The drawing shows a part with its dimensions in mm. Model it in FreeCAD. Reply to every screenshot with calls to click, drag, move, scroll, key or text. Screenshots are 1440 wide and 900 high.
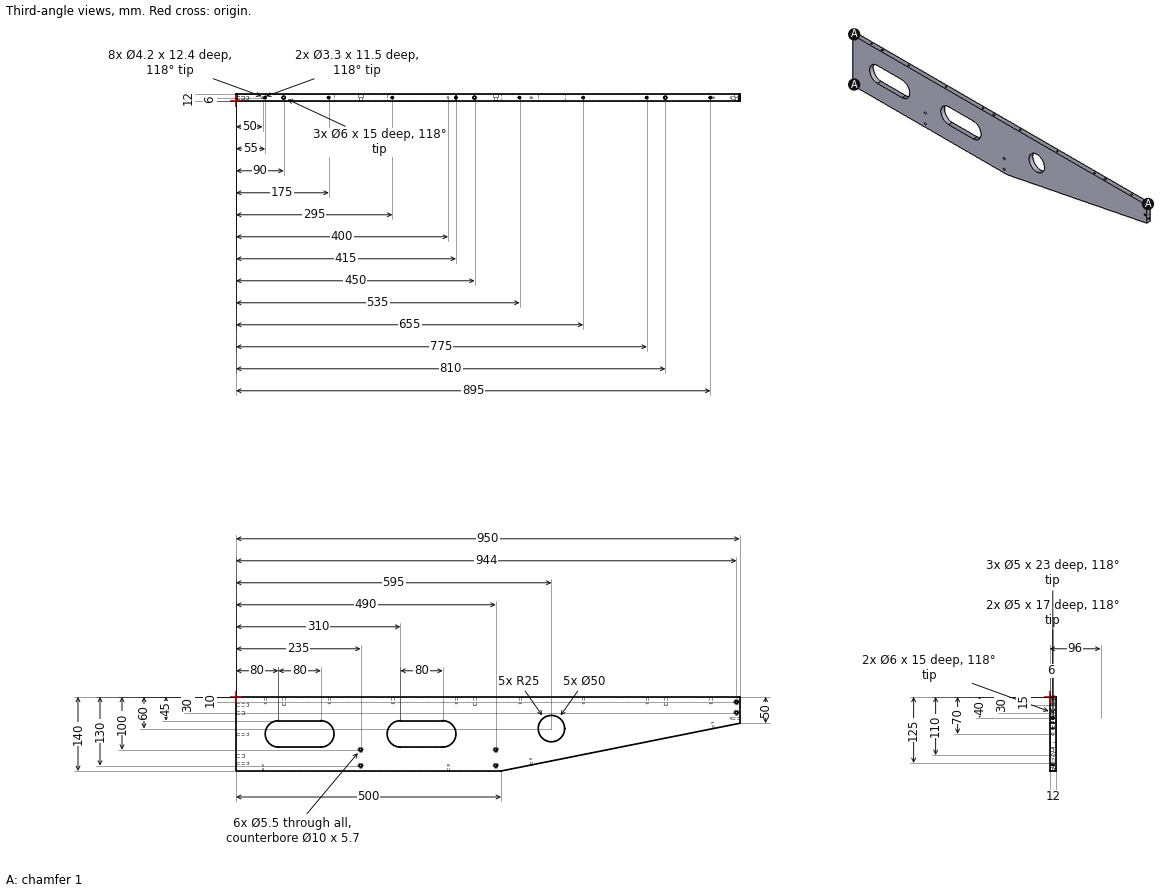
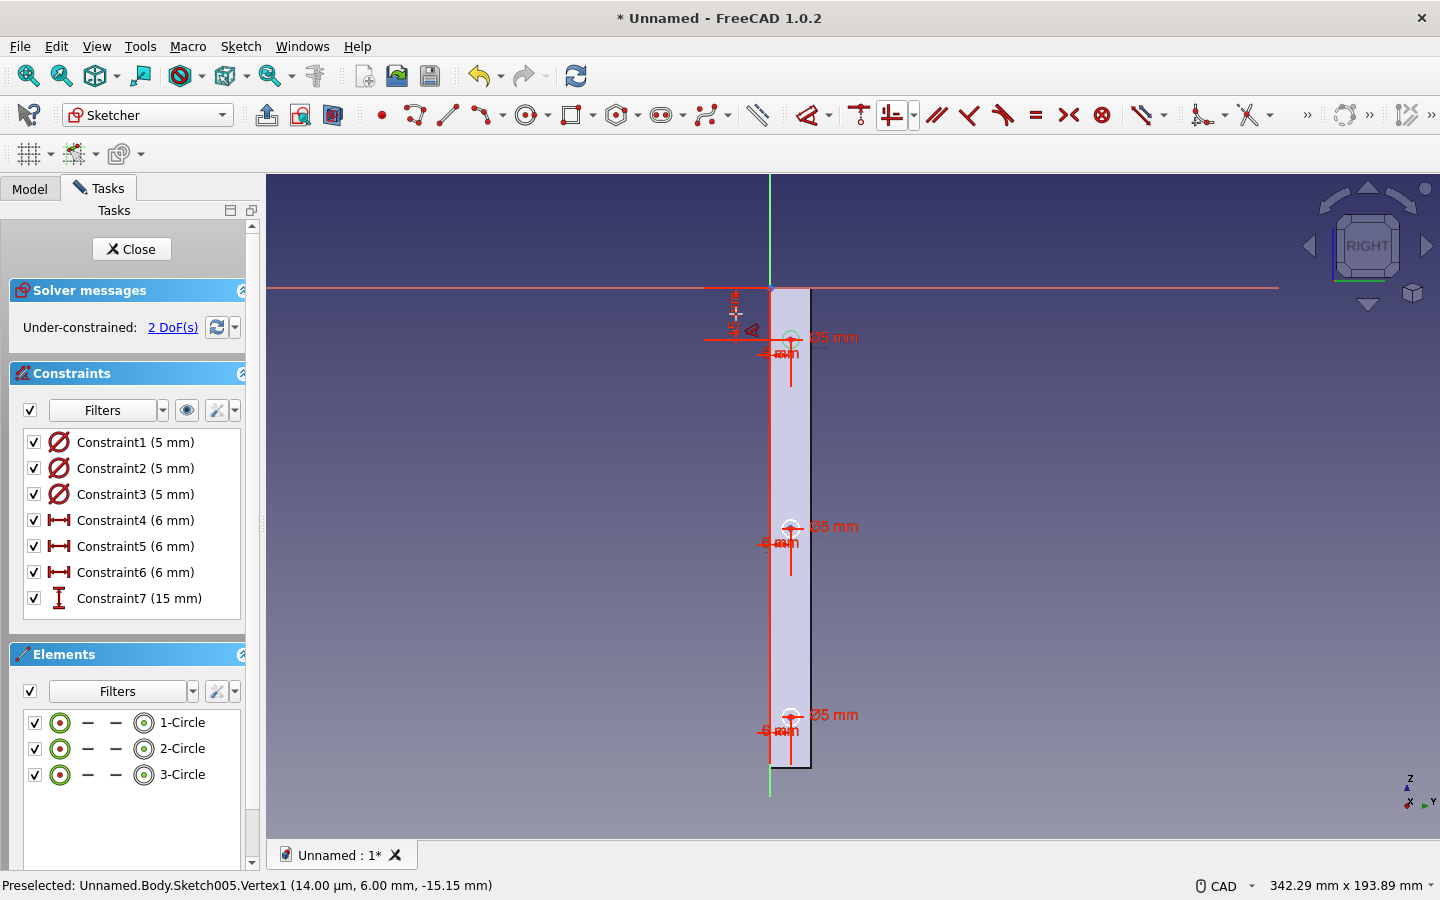
click(791, 529)
click(736, 408)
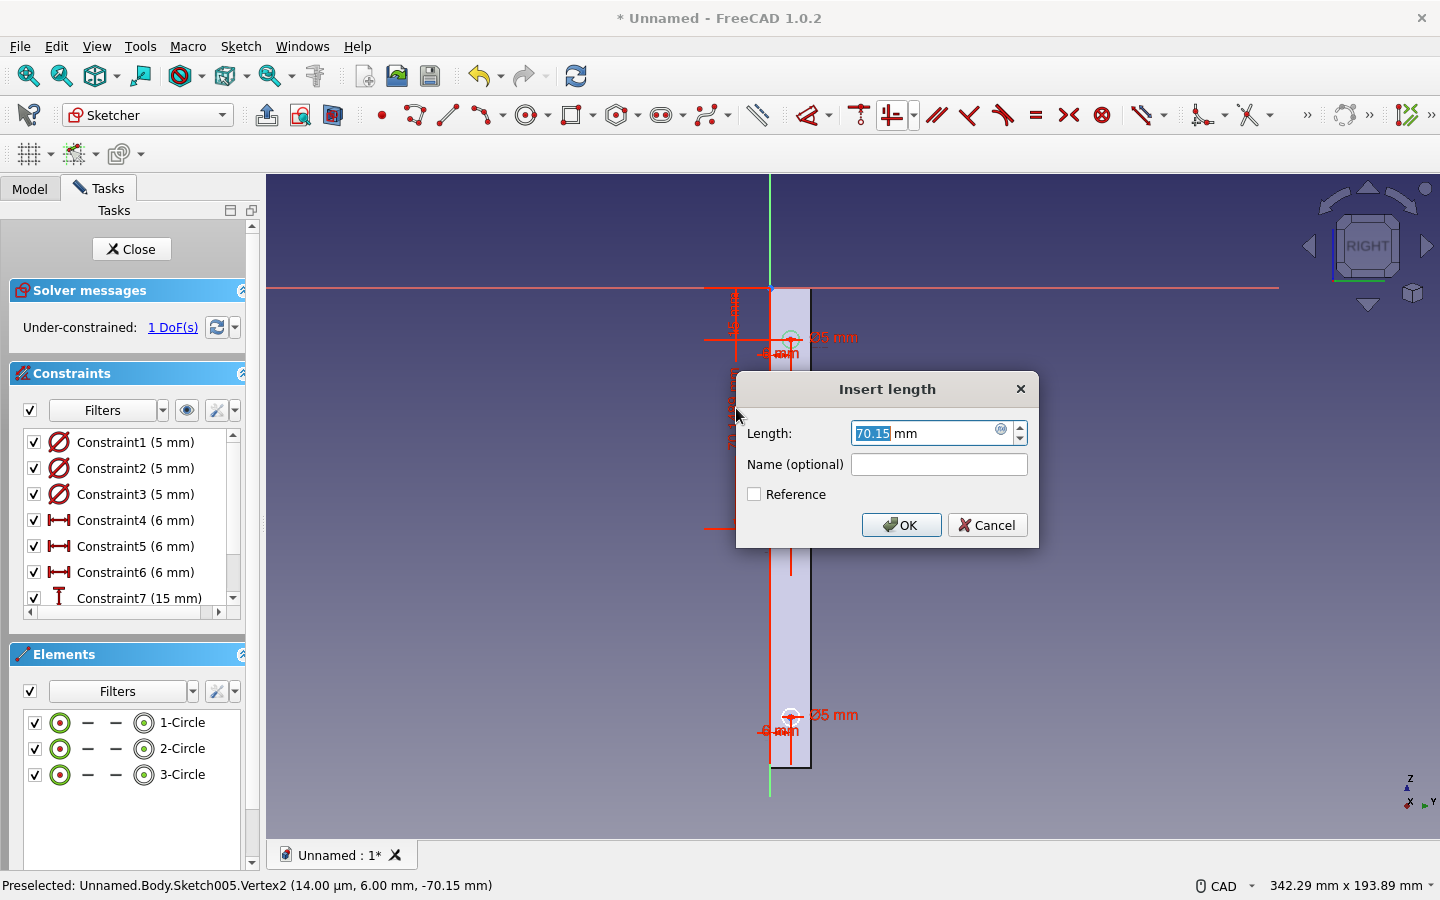
text(70)
key(Return)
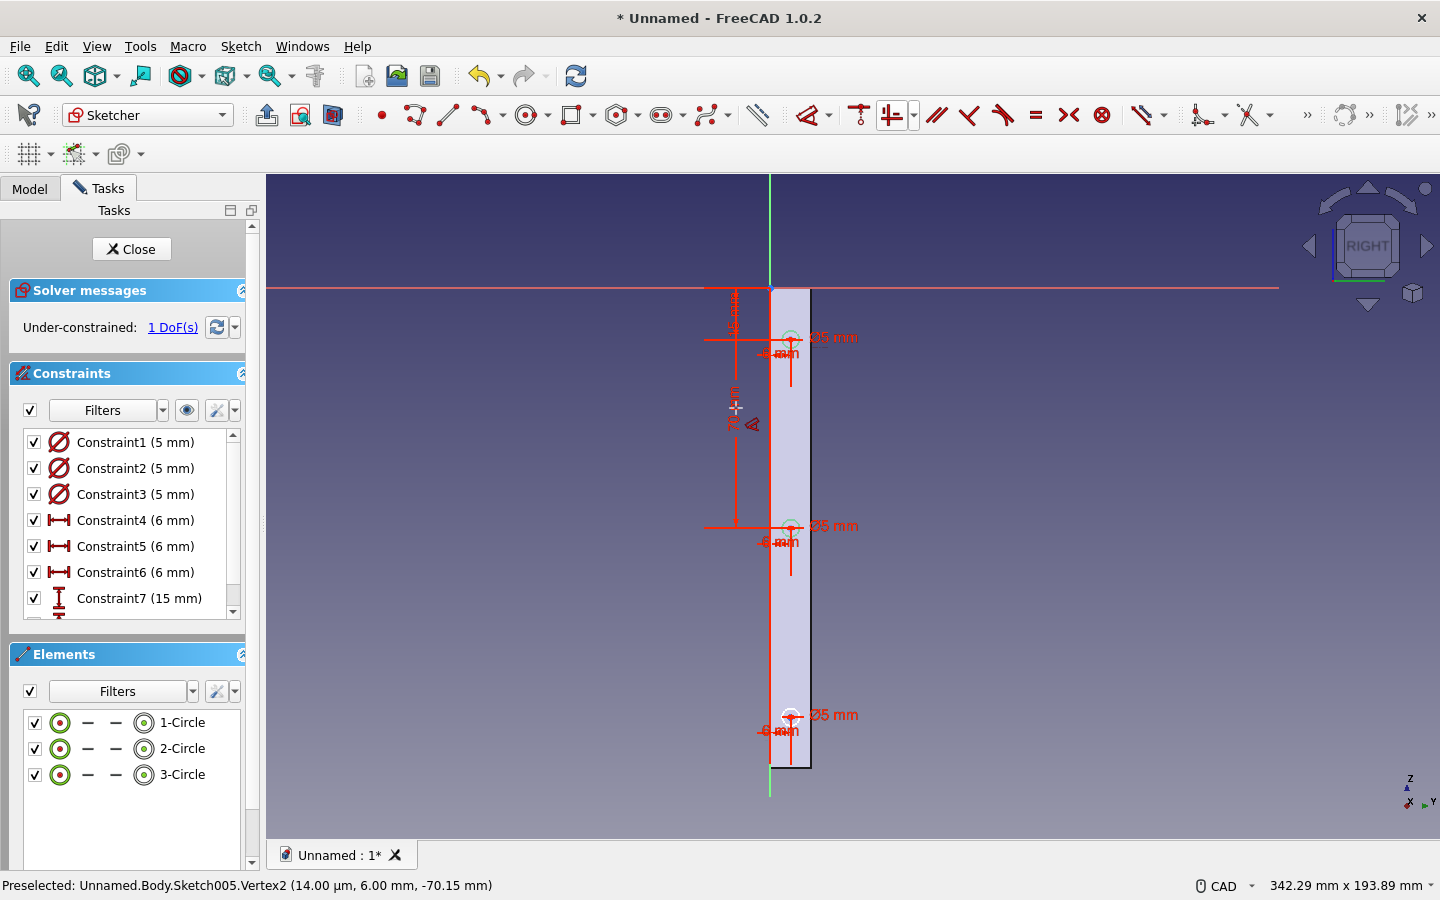
click(791, 717)
click(736, 503)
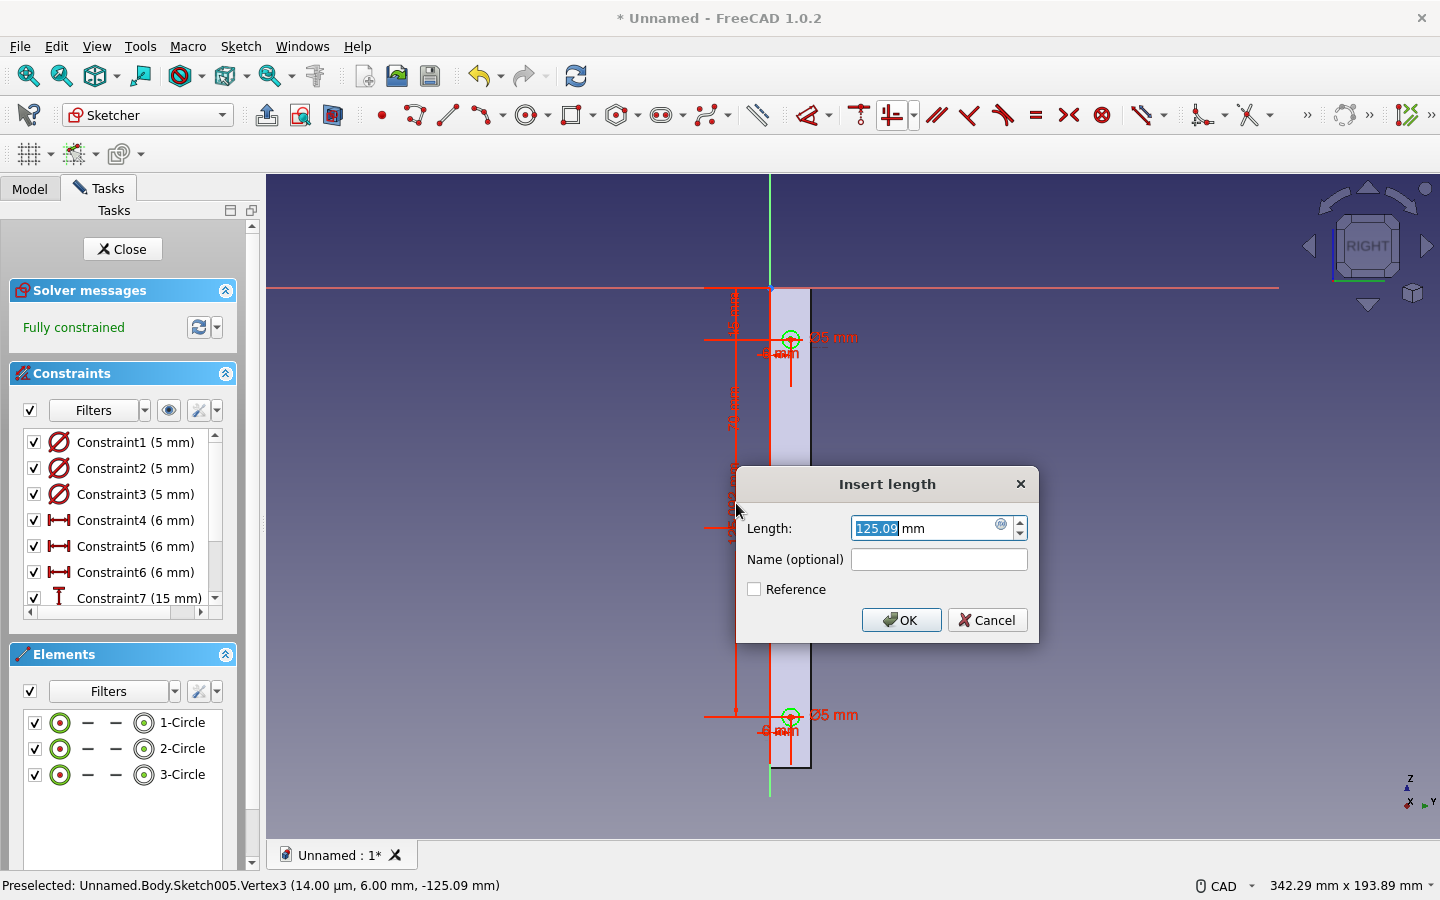
text(125)
key(Return)
key(Escape)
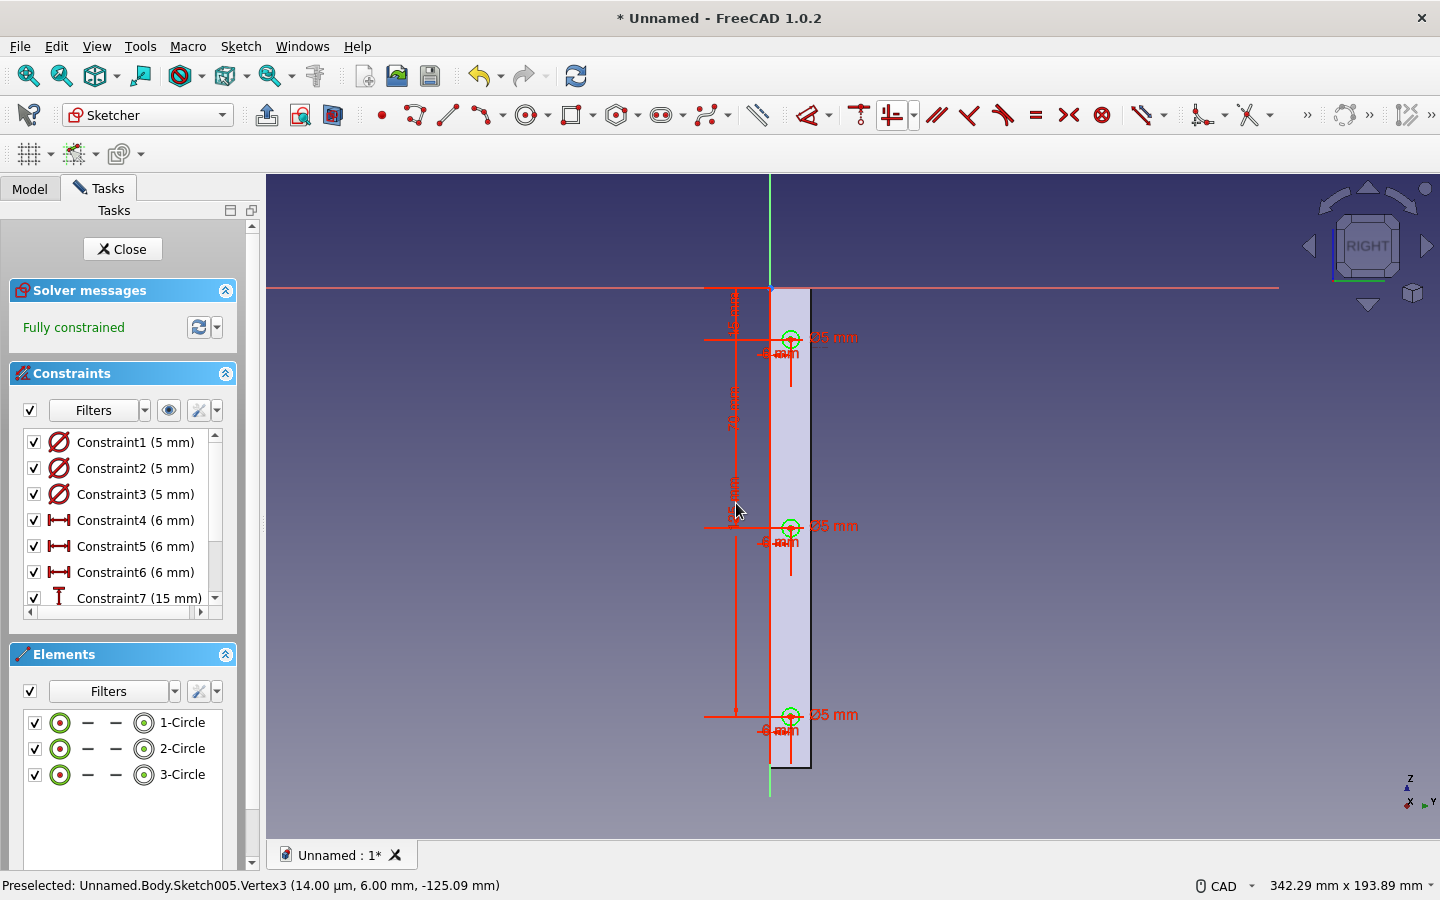
click(123, 249)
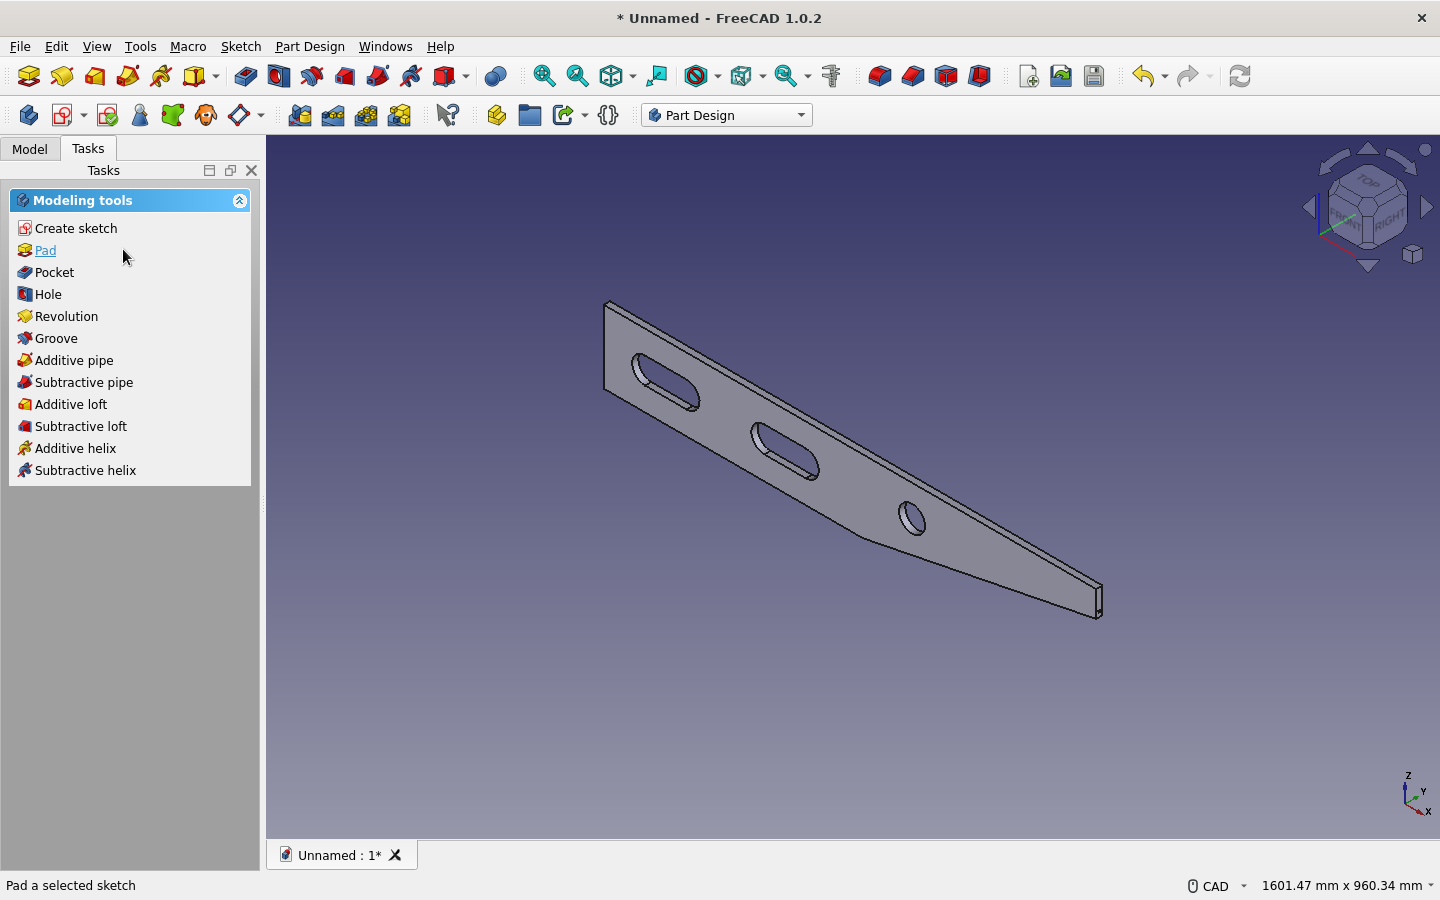
click(279, 76)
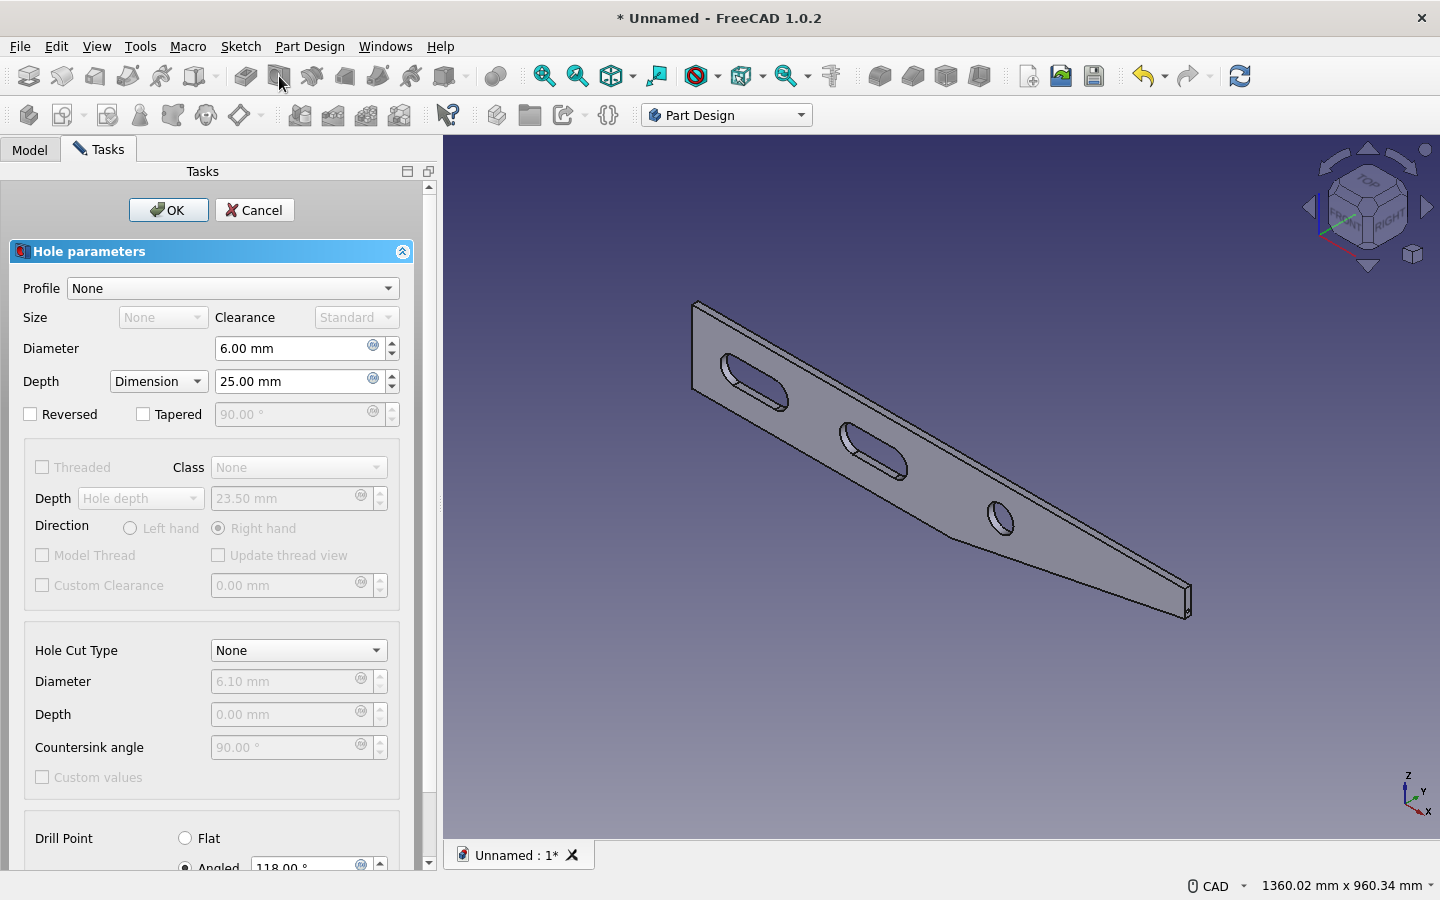
triple_click(300, 348)